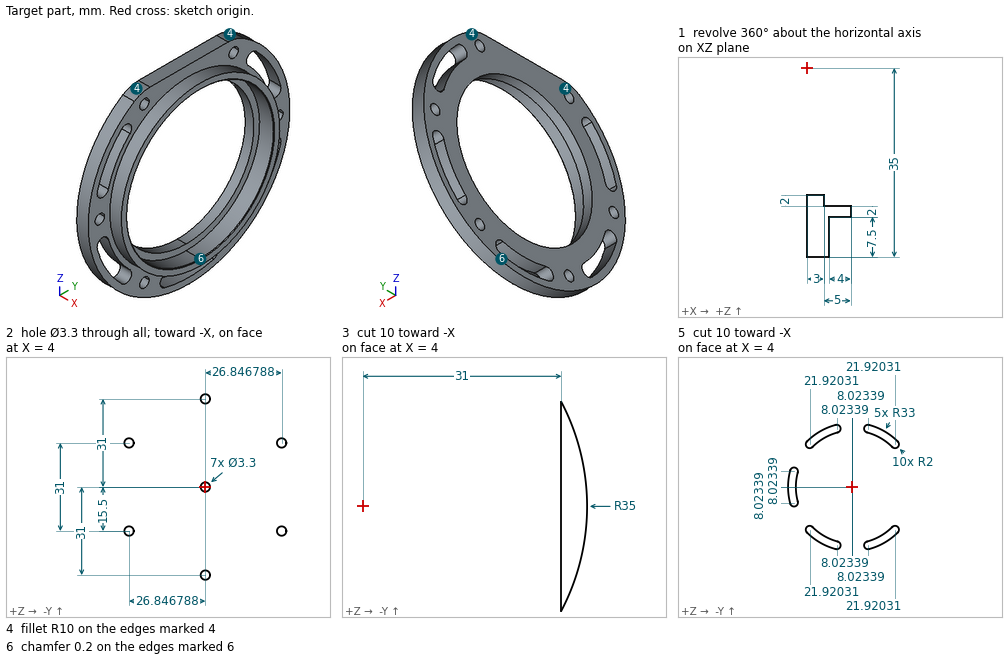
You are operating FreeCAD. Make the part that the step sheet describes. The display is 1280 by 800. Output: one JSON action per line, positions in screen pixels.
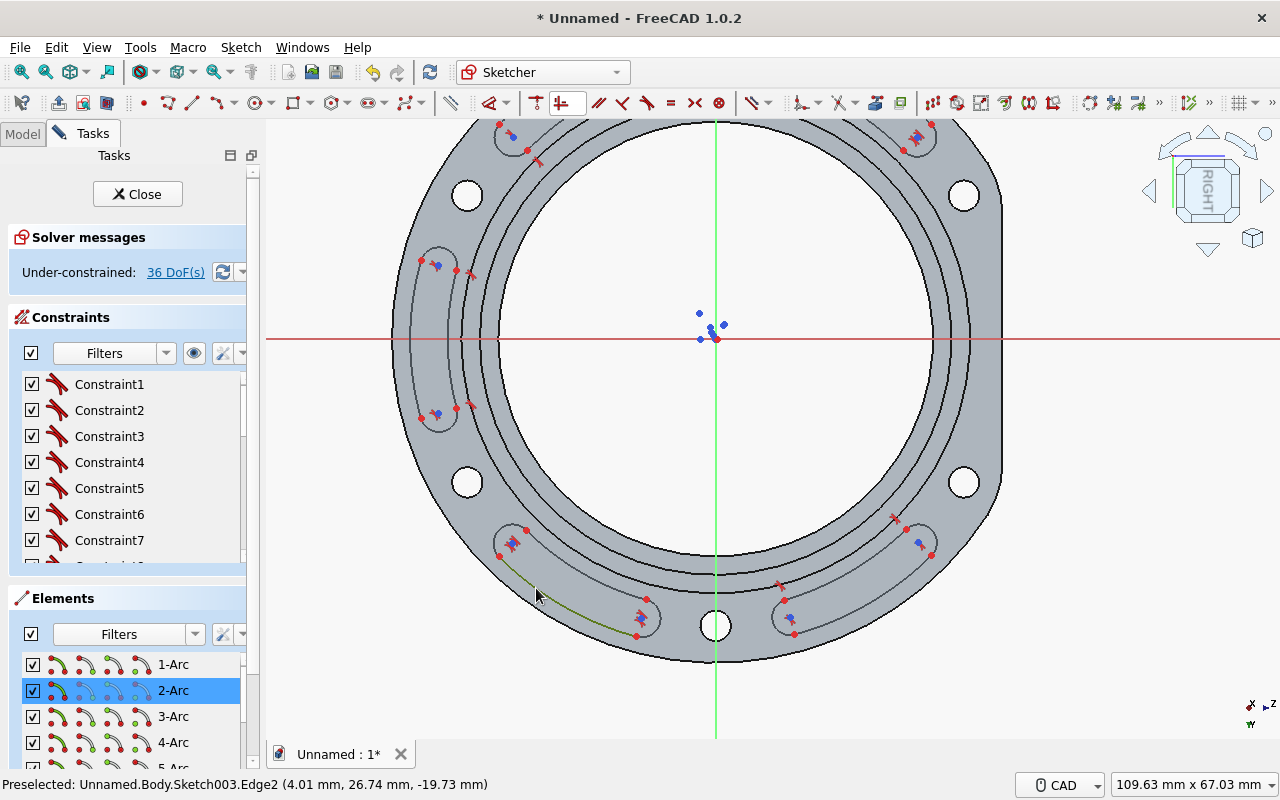
{"action": "left_click", "coordinate": [412, 308]}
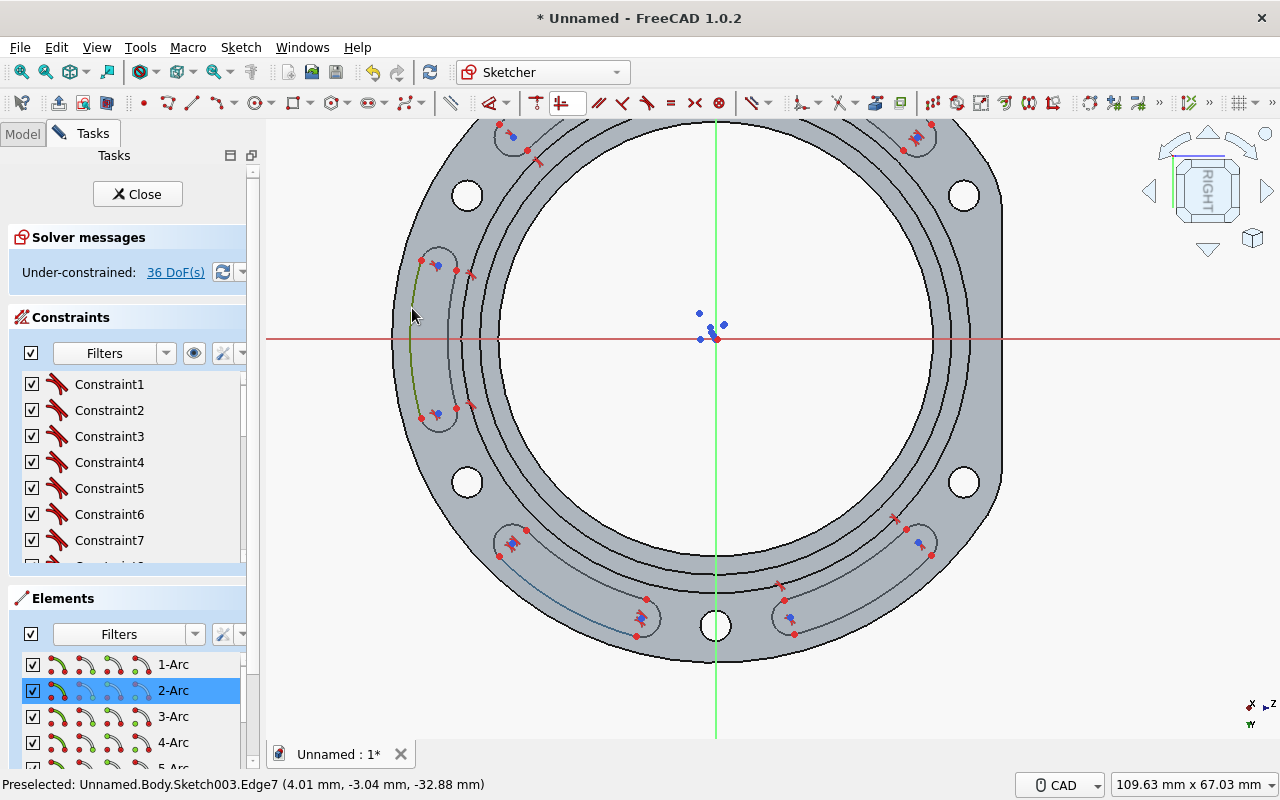
{"action": "left_click", "coordinate": [536, 104]}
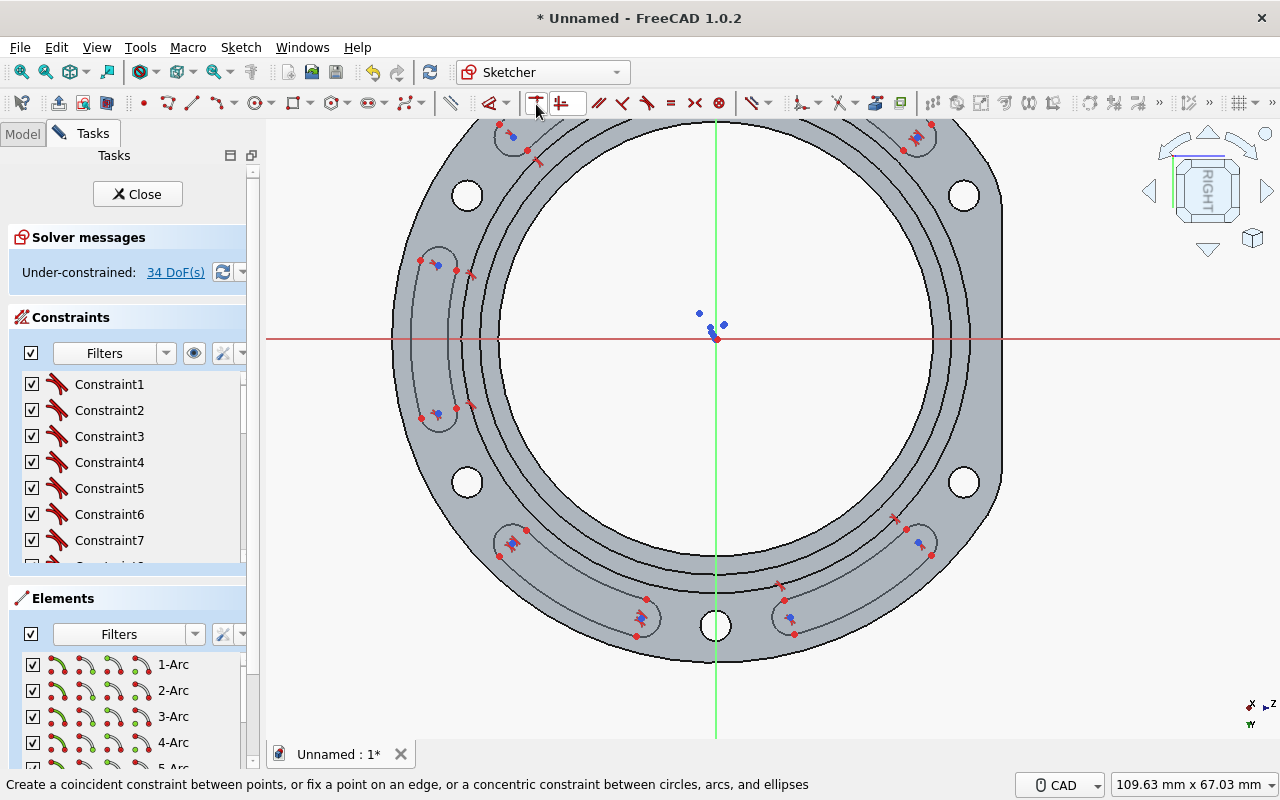
{"action": "left_click", "coordinate": [536, 588]}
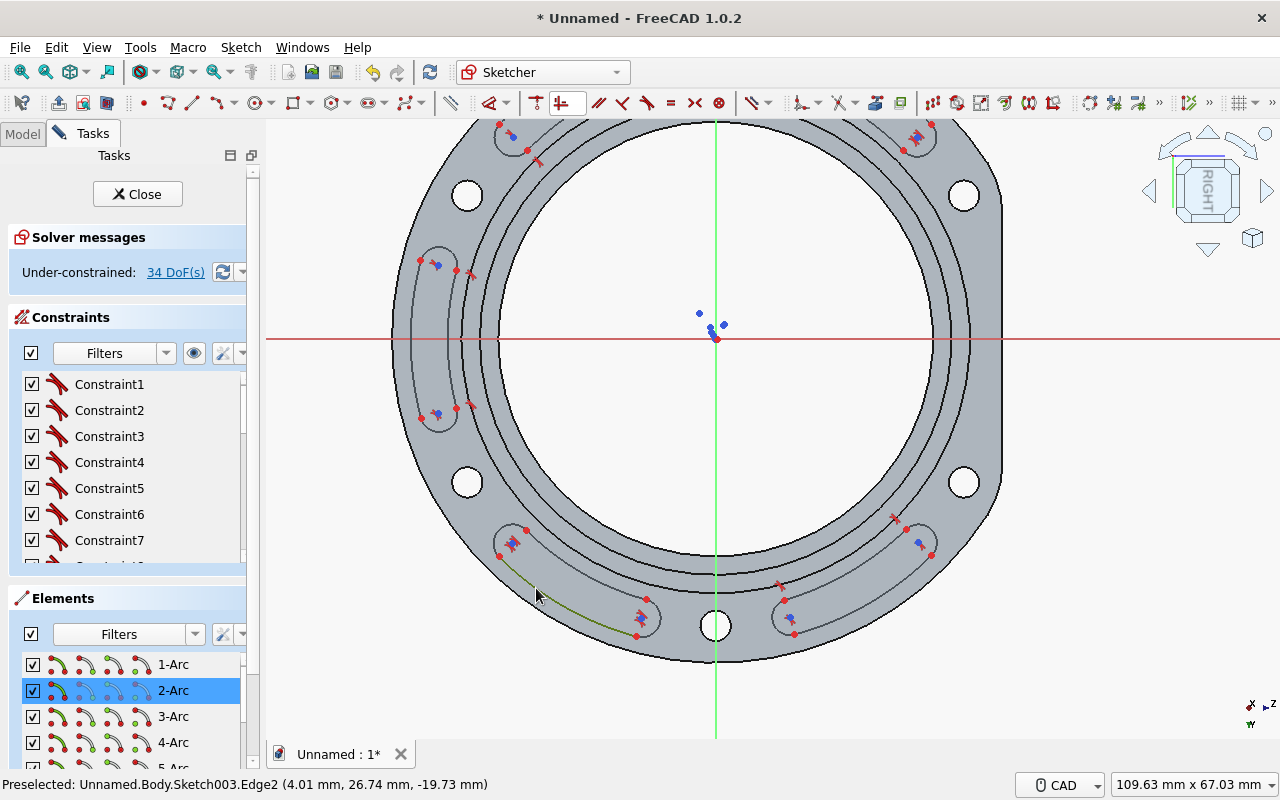
{"action": "scroll", "coordinate": [773, 612], "scroll_direction": "down", "scroll_amount": 2}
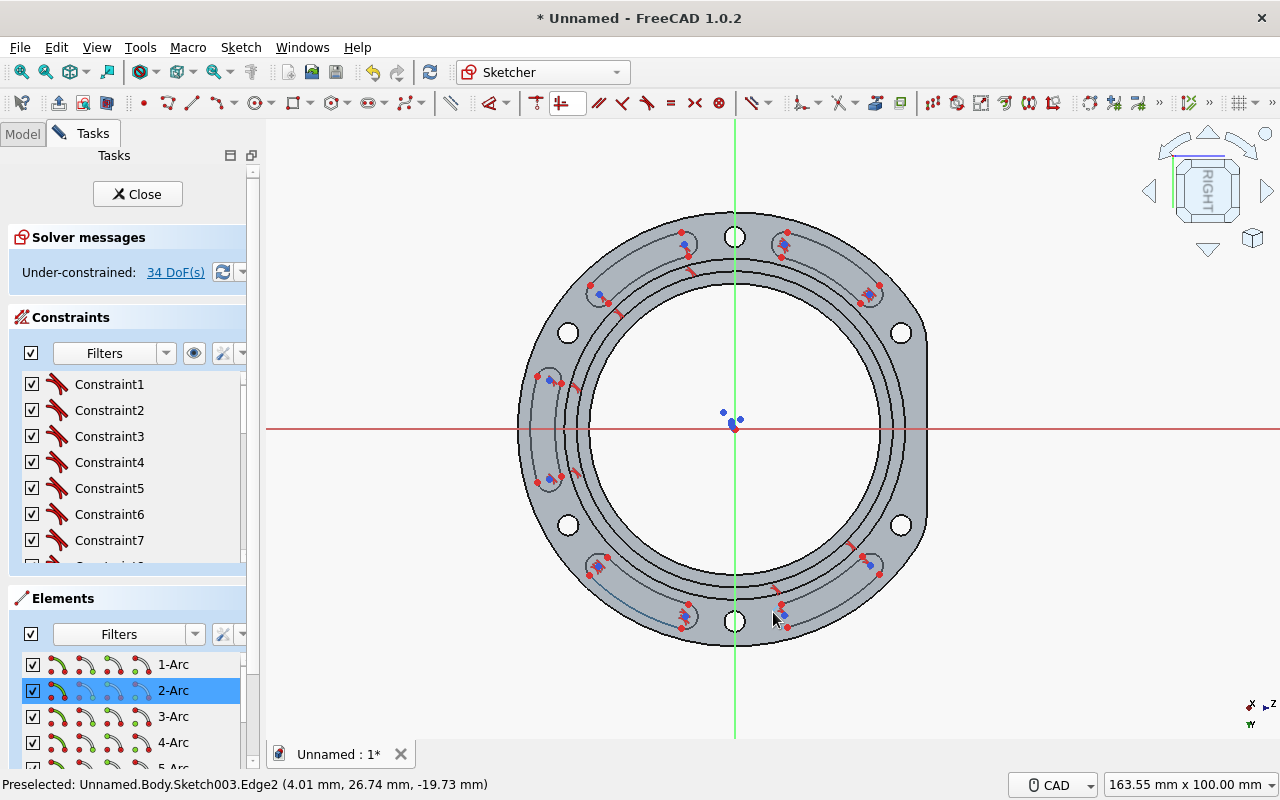
{"action": "left_click", "coordinate": [662, 266]}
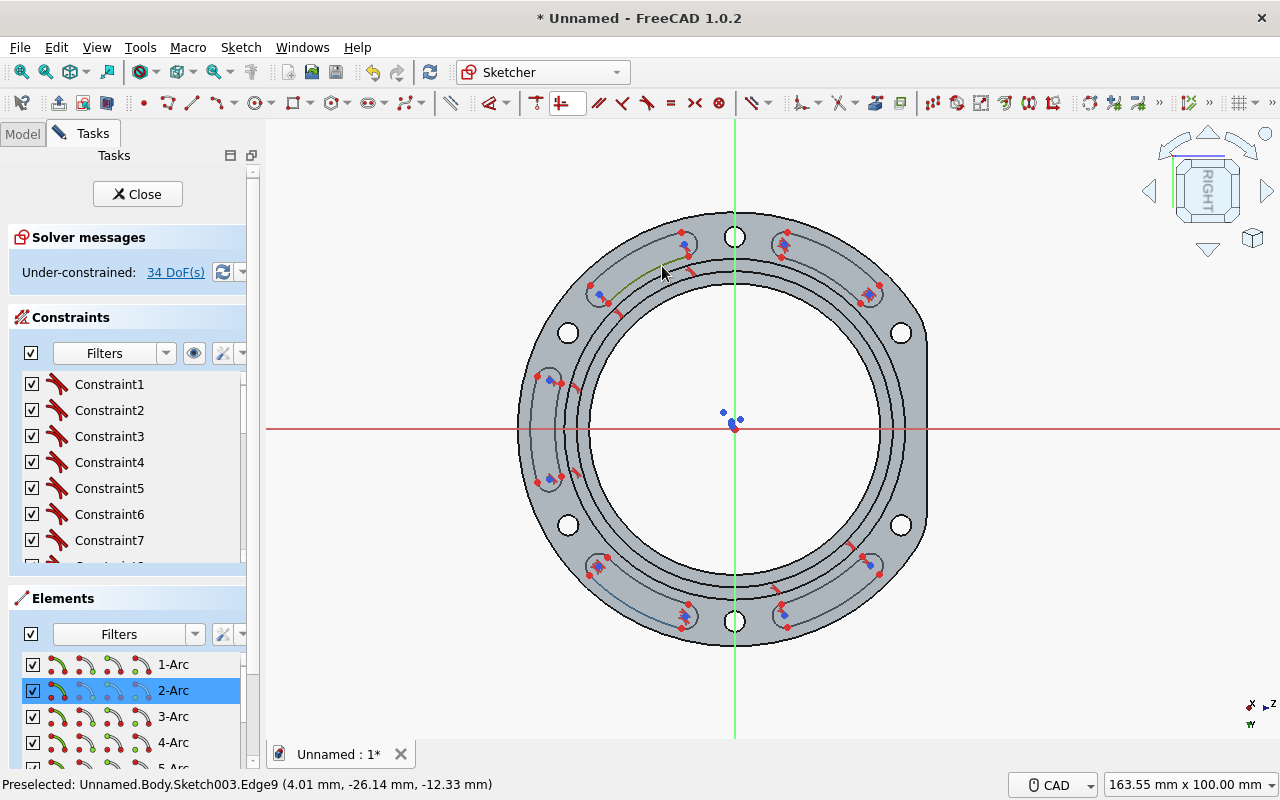
{"action": "left_click", "coordinate": [536, 104]}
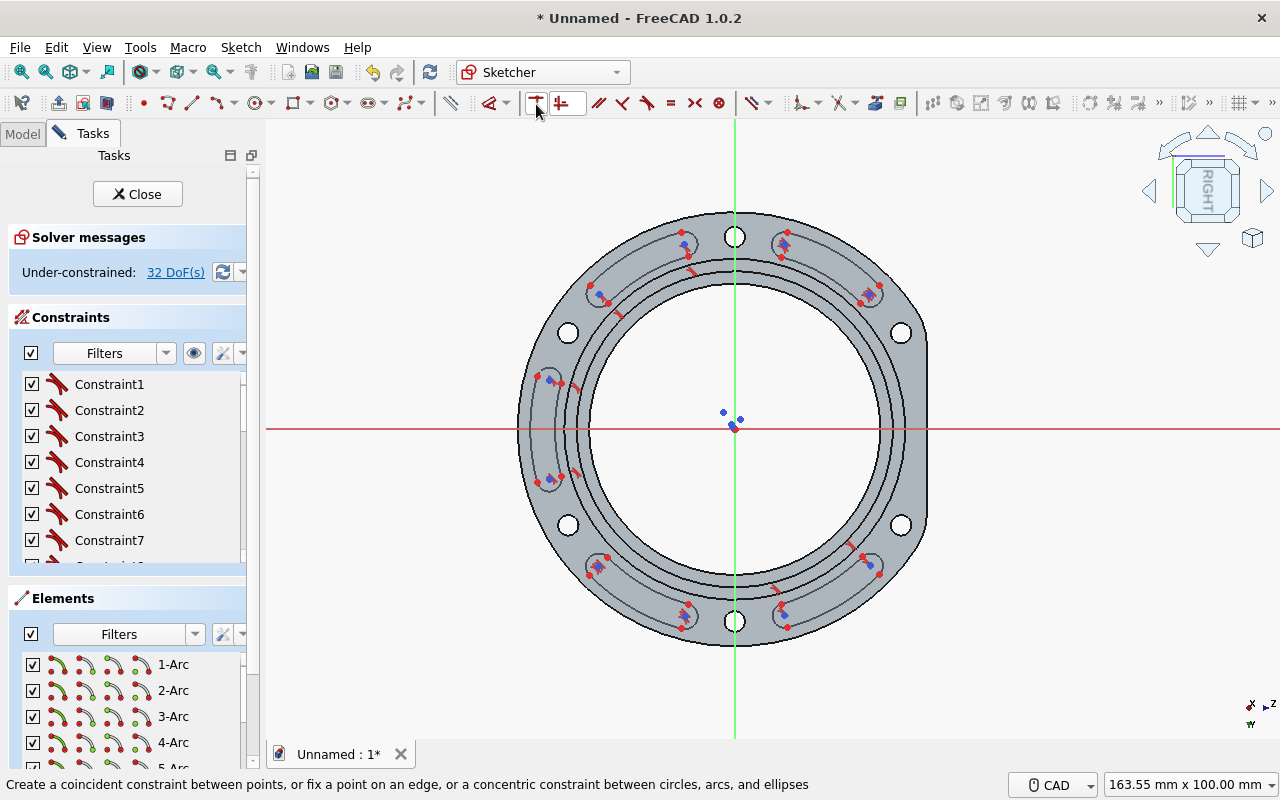
{"action": "left_click", "coordinate": [614, 596]}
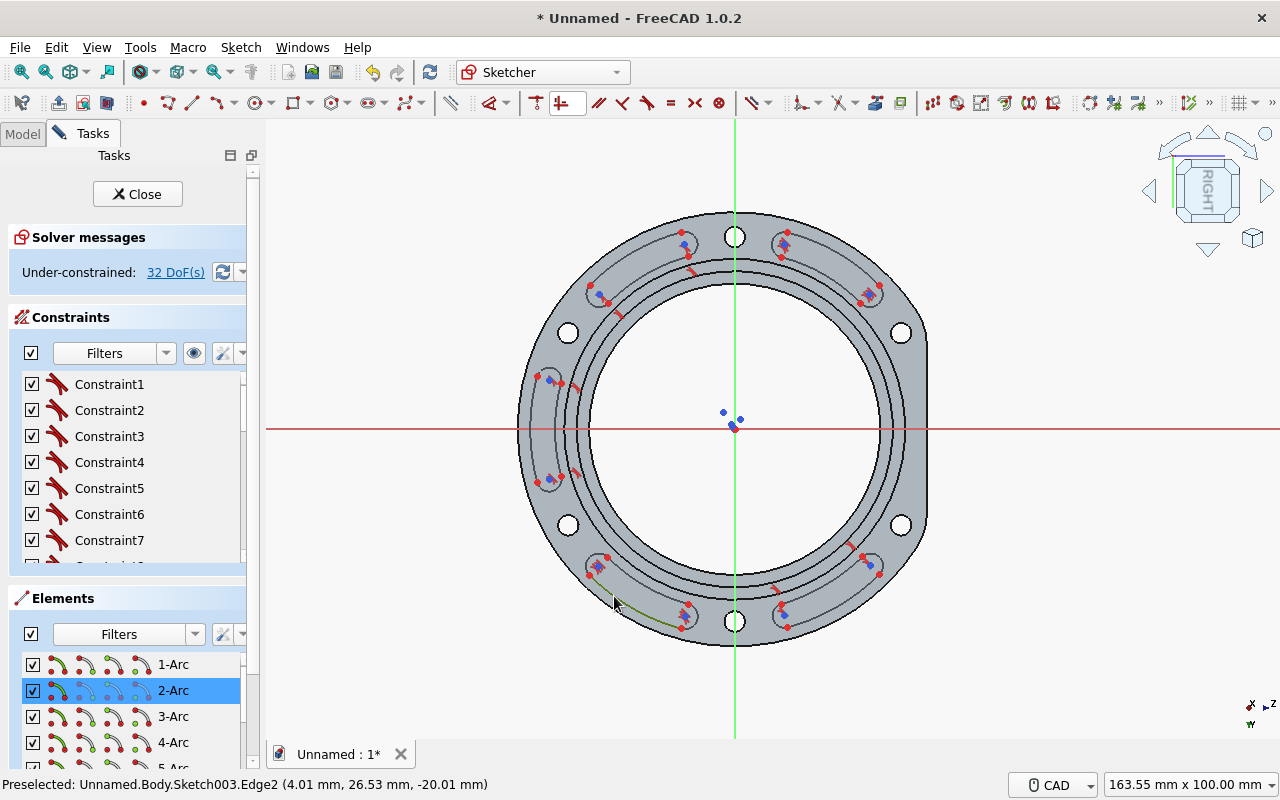
{"action": "left_click", "coordinate": [651, 243]}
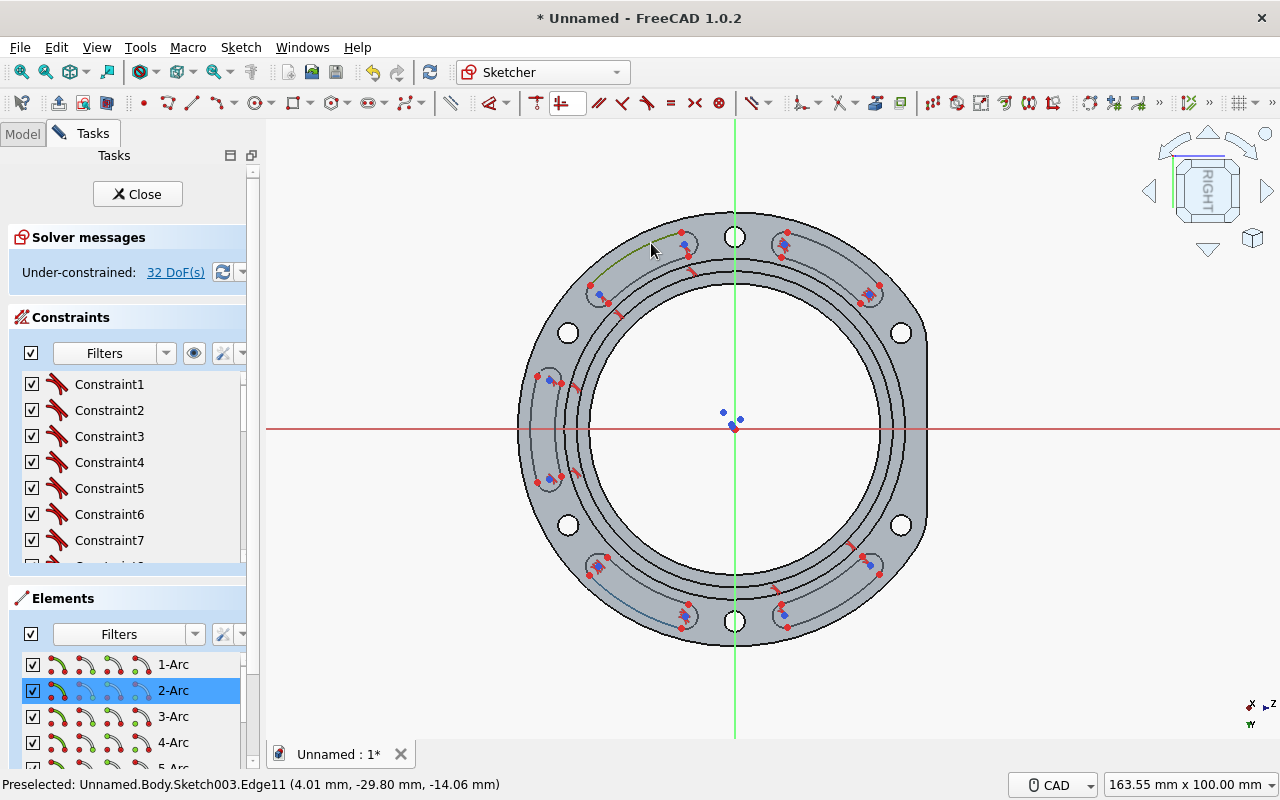
{"action": "left_click", "coordinate": [536, 104]}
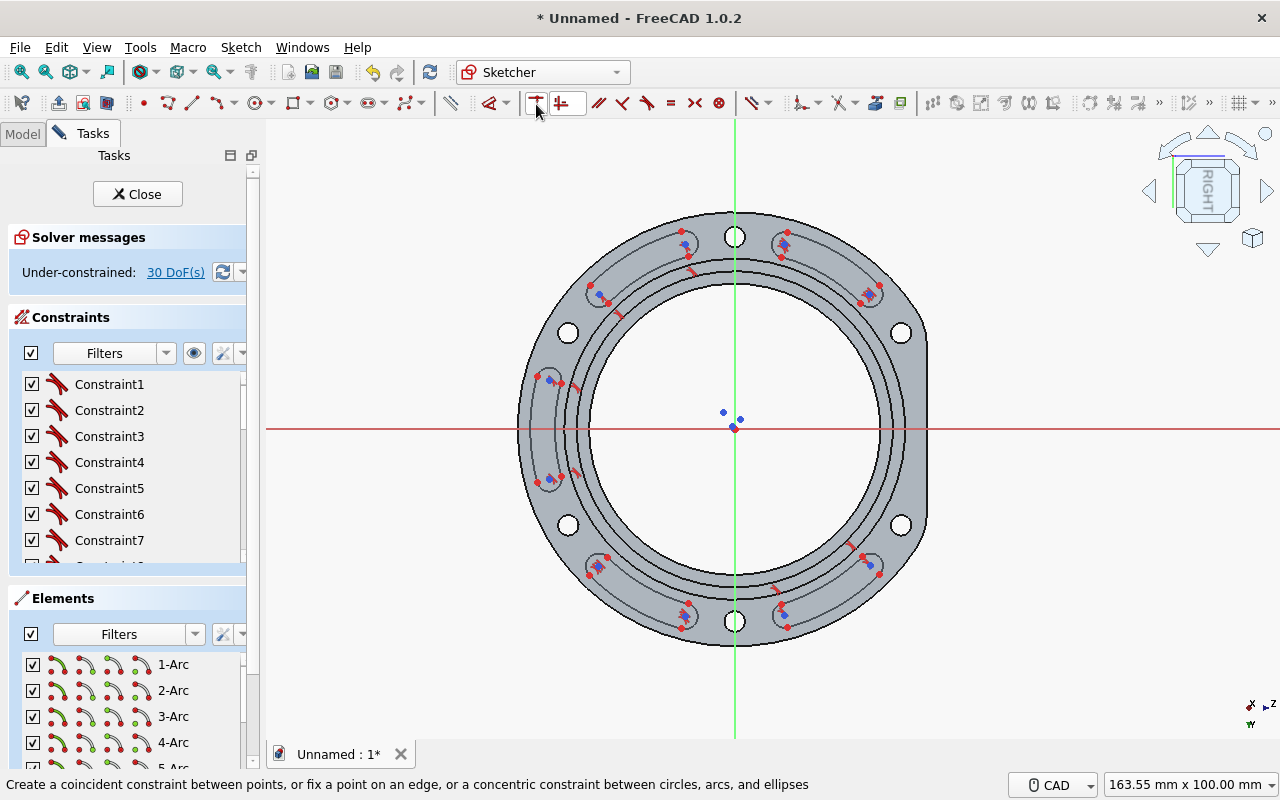
{"action": "left_click", "coordinate": [614, 596]}